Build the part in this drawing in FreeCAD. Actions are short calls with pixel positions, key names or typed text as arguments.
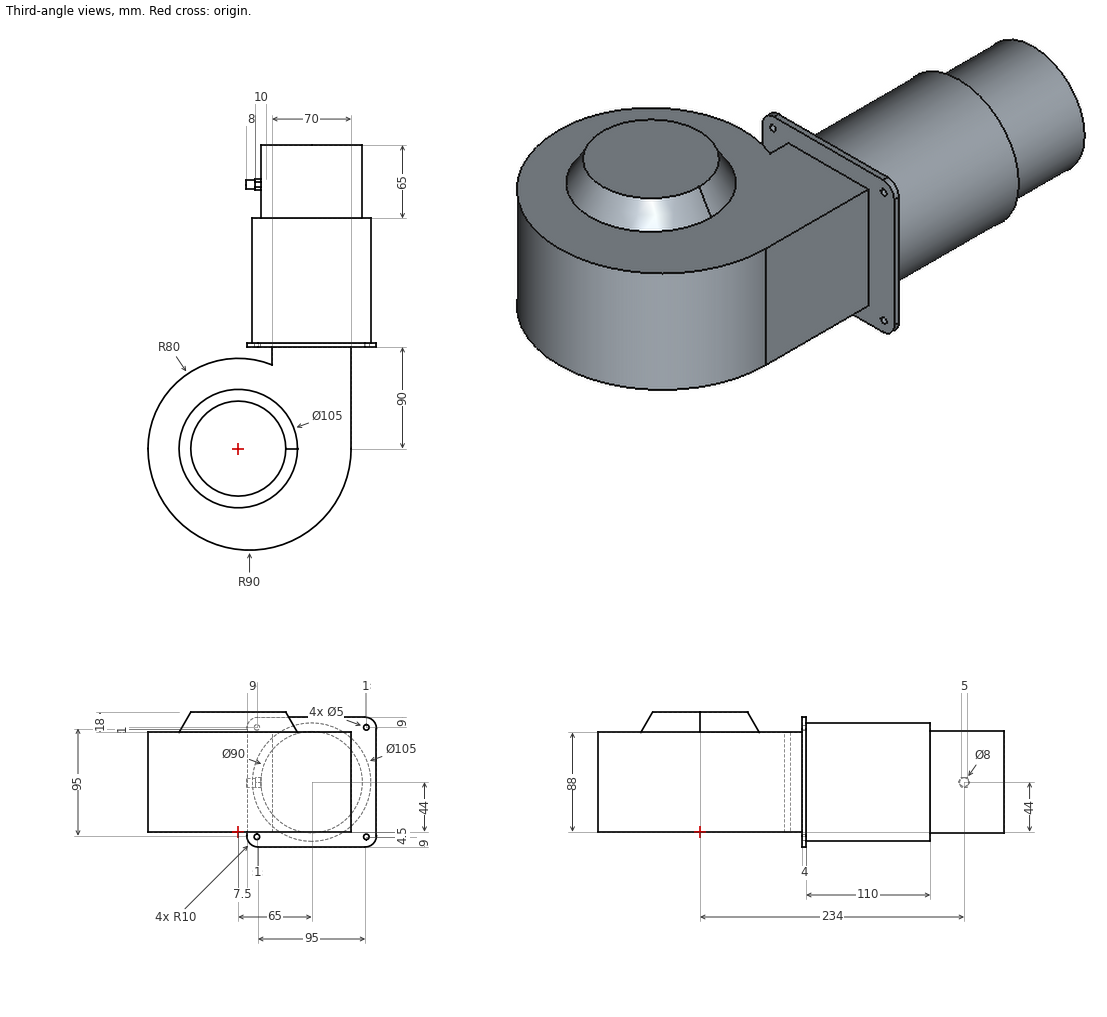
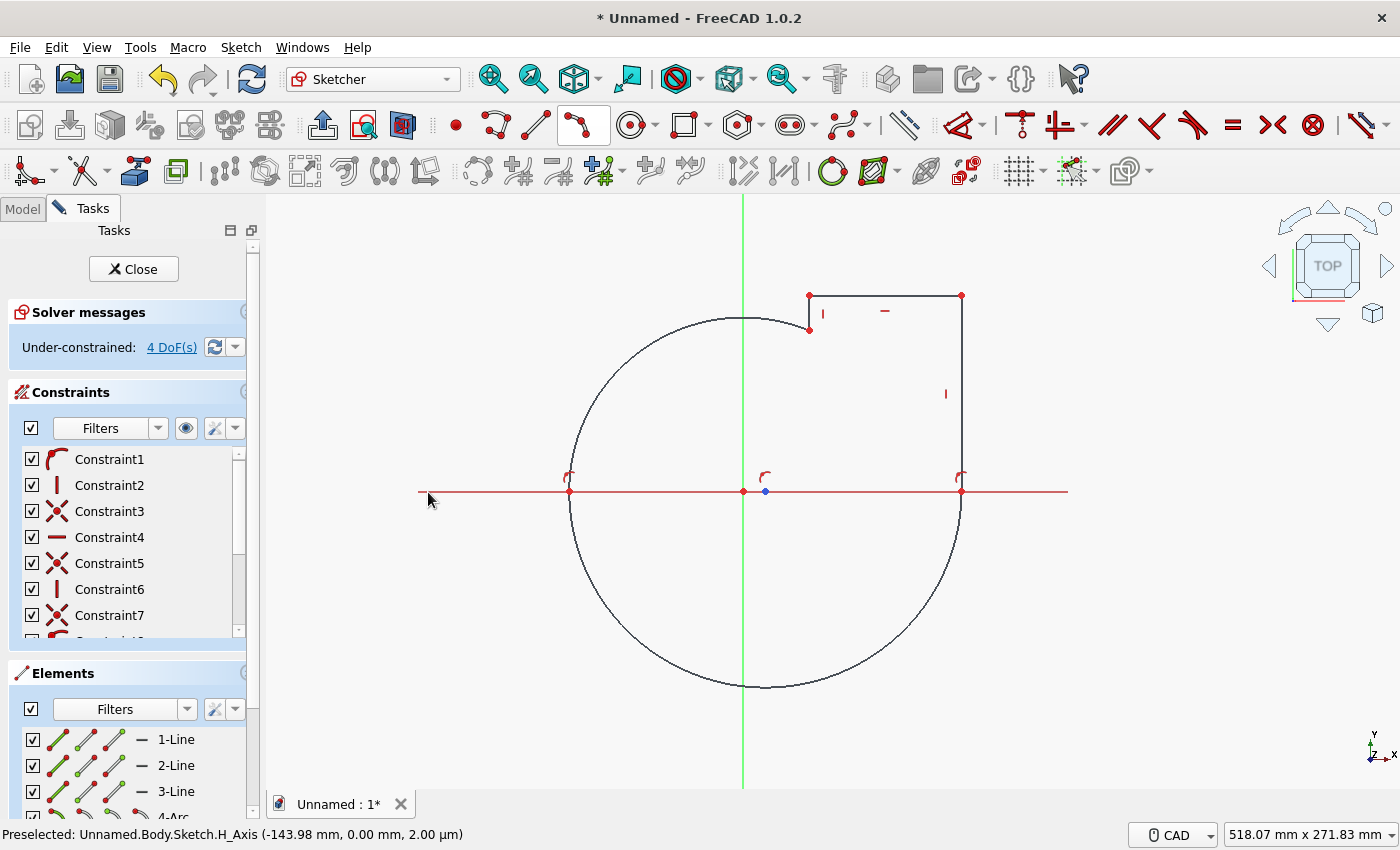
click(958, 126)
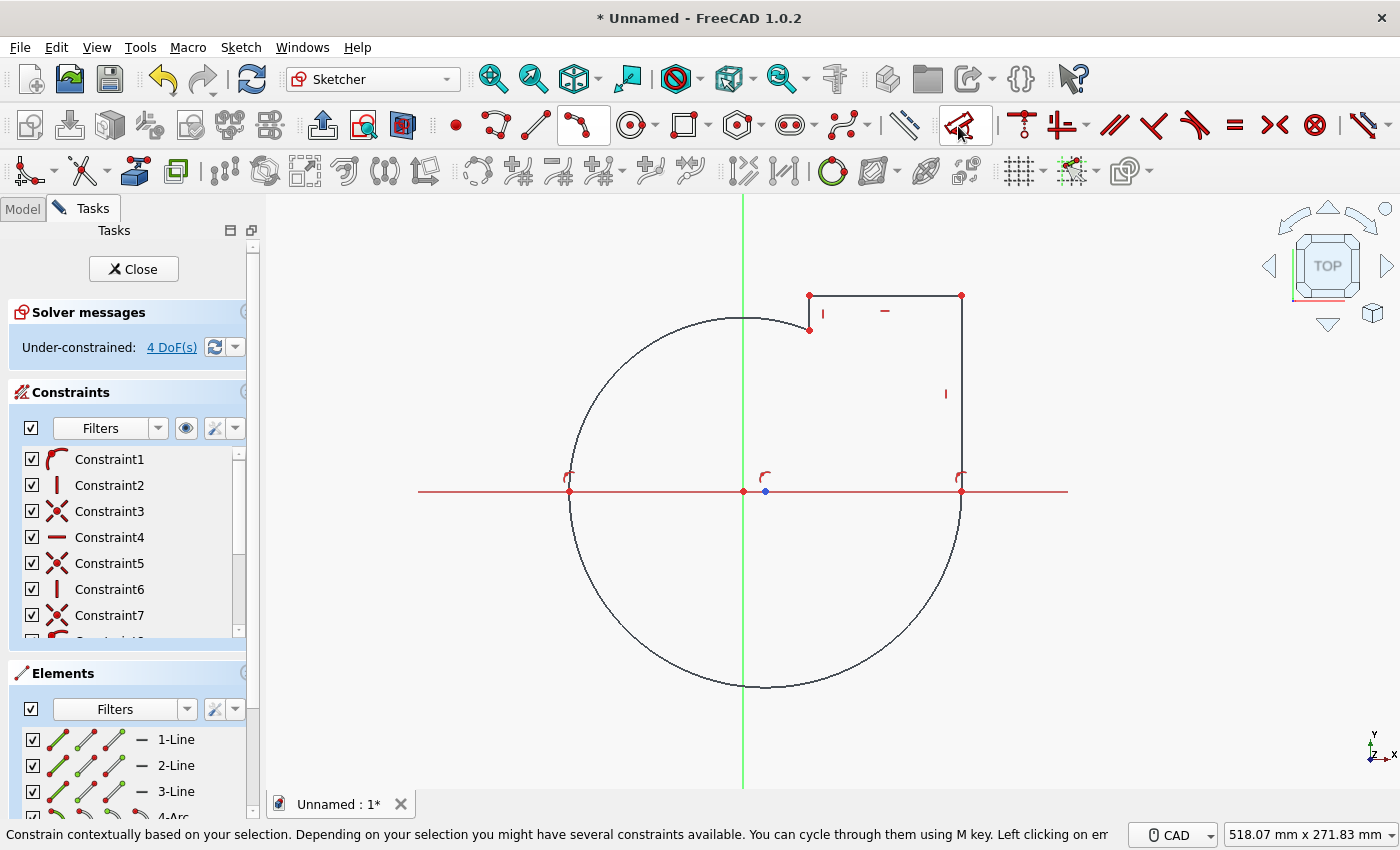
click(709, 321)
click(703, 290)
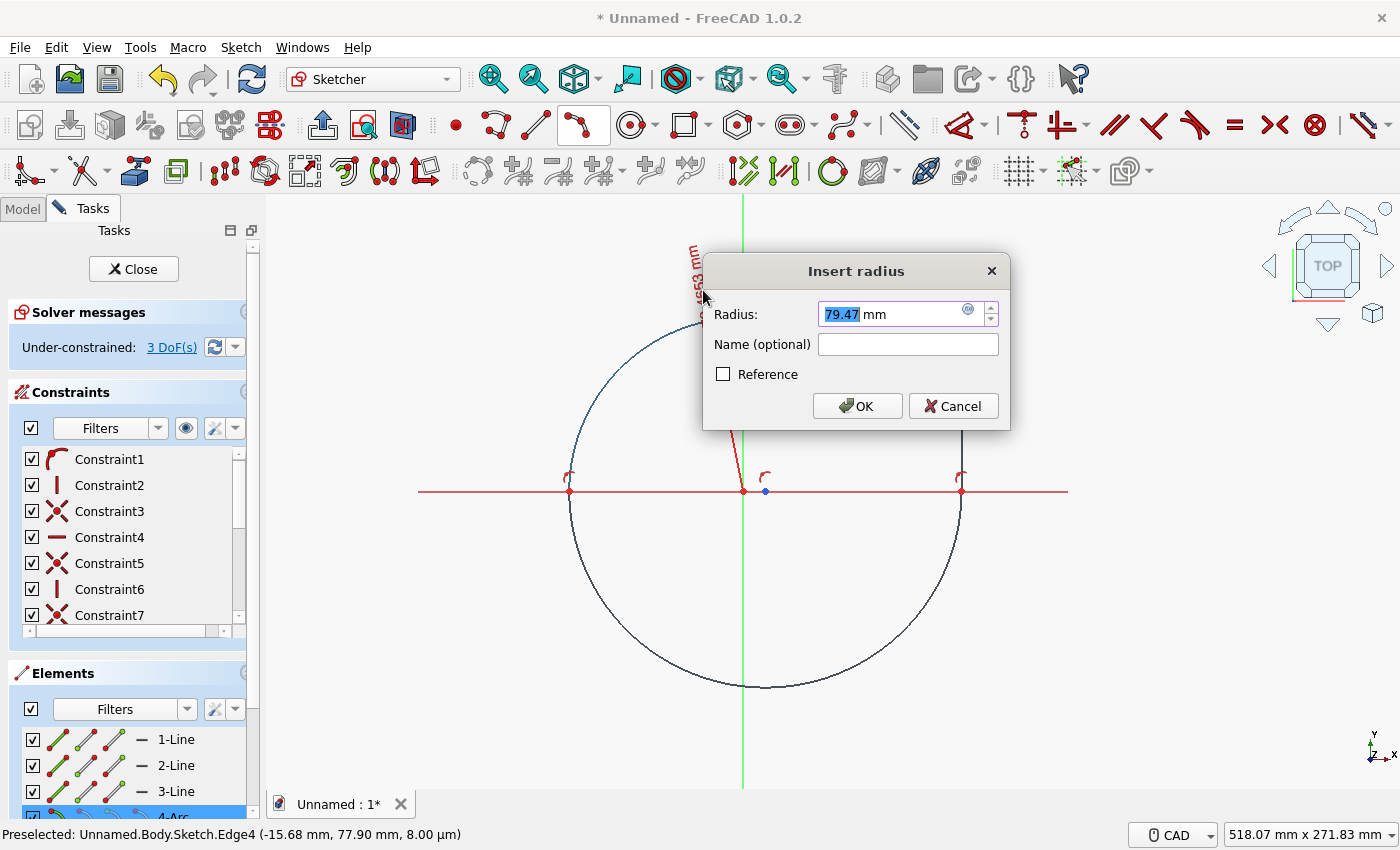
text(80)
key(Return)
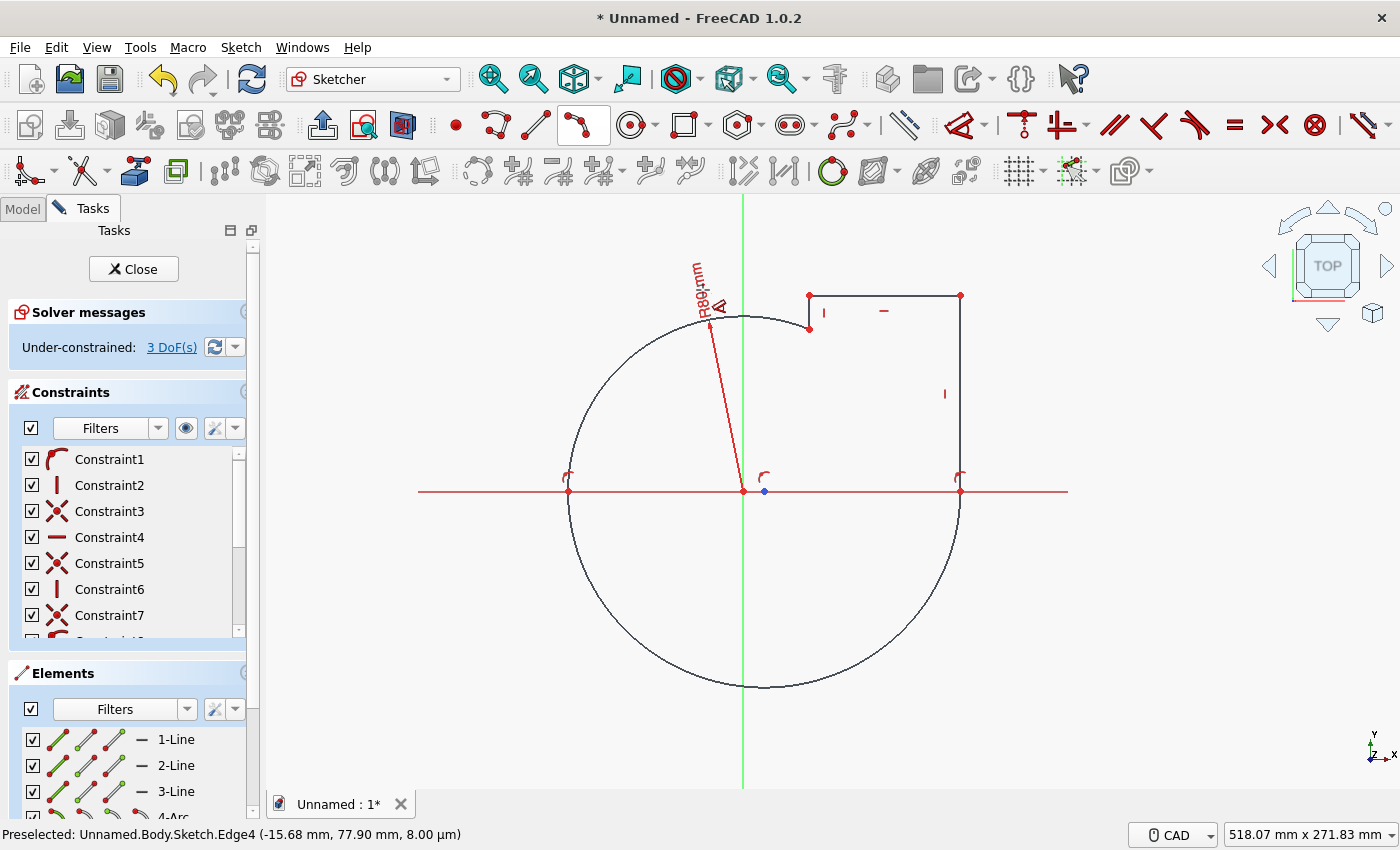
click(649, 650)
click(630, 676)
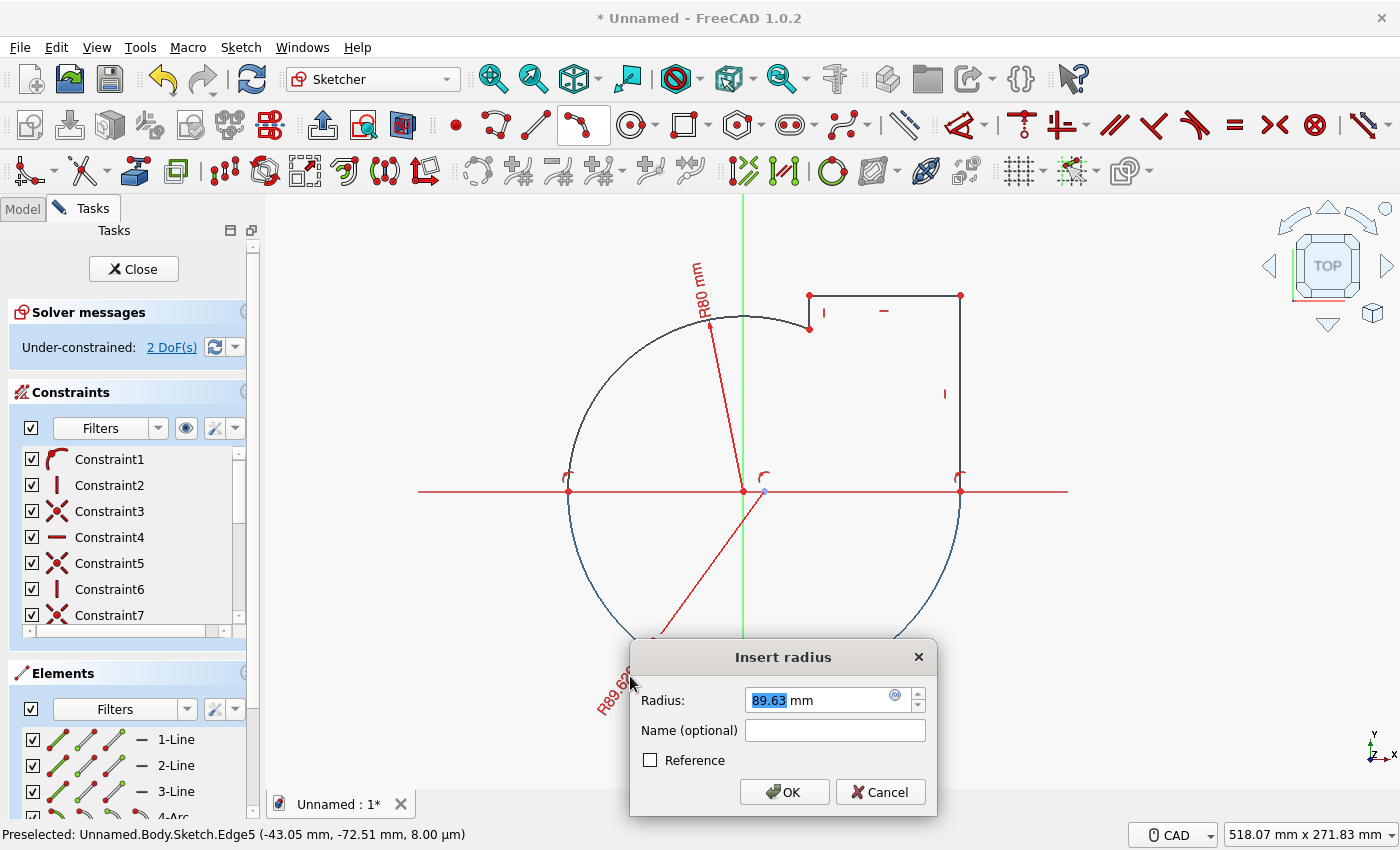
text(90)
key(Return)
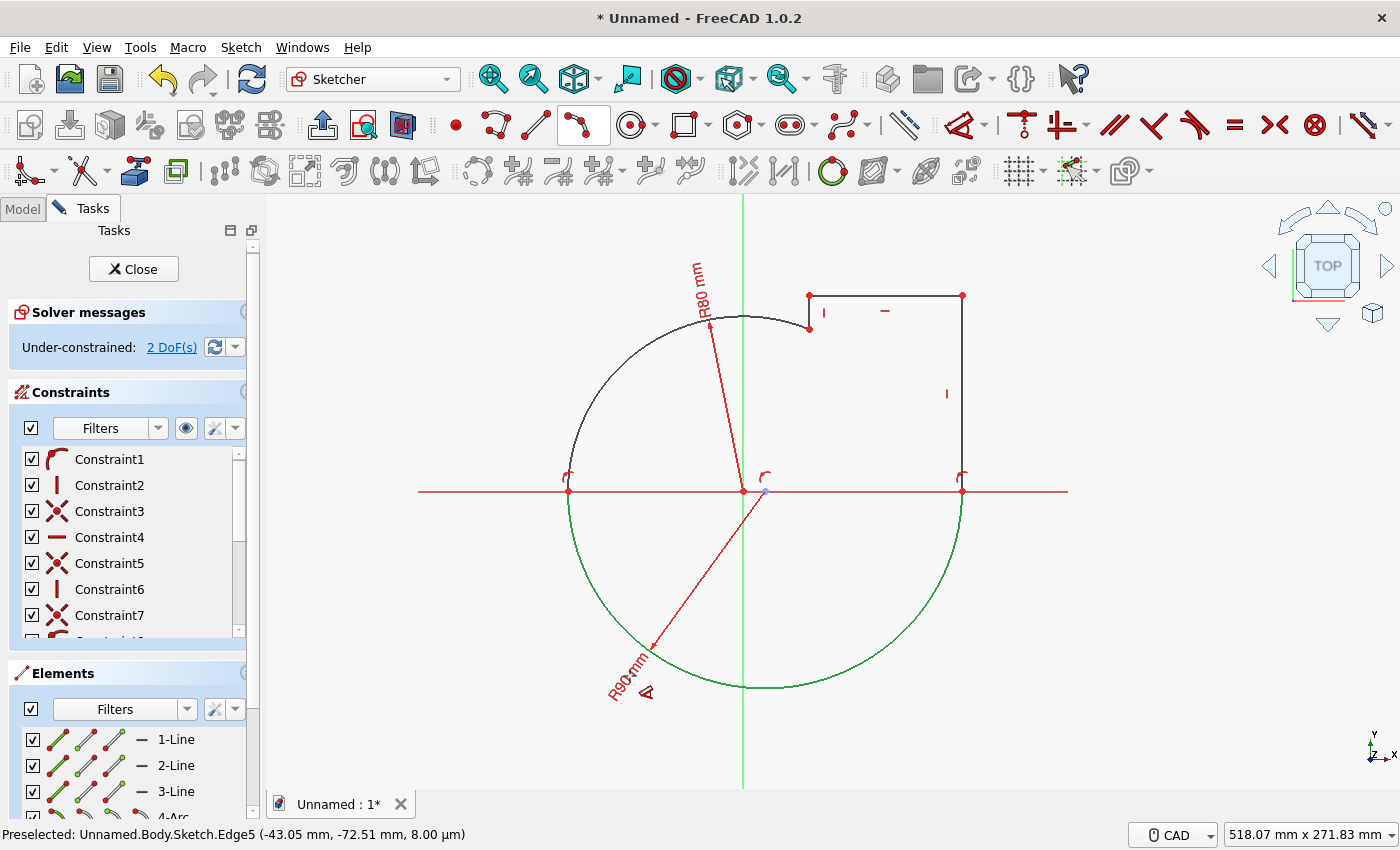
click(962, 433)
click(996, 394)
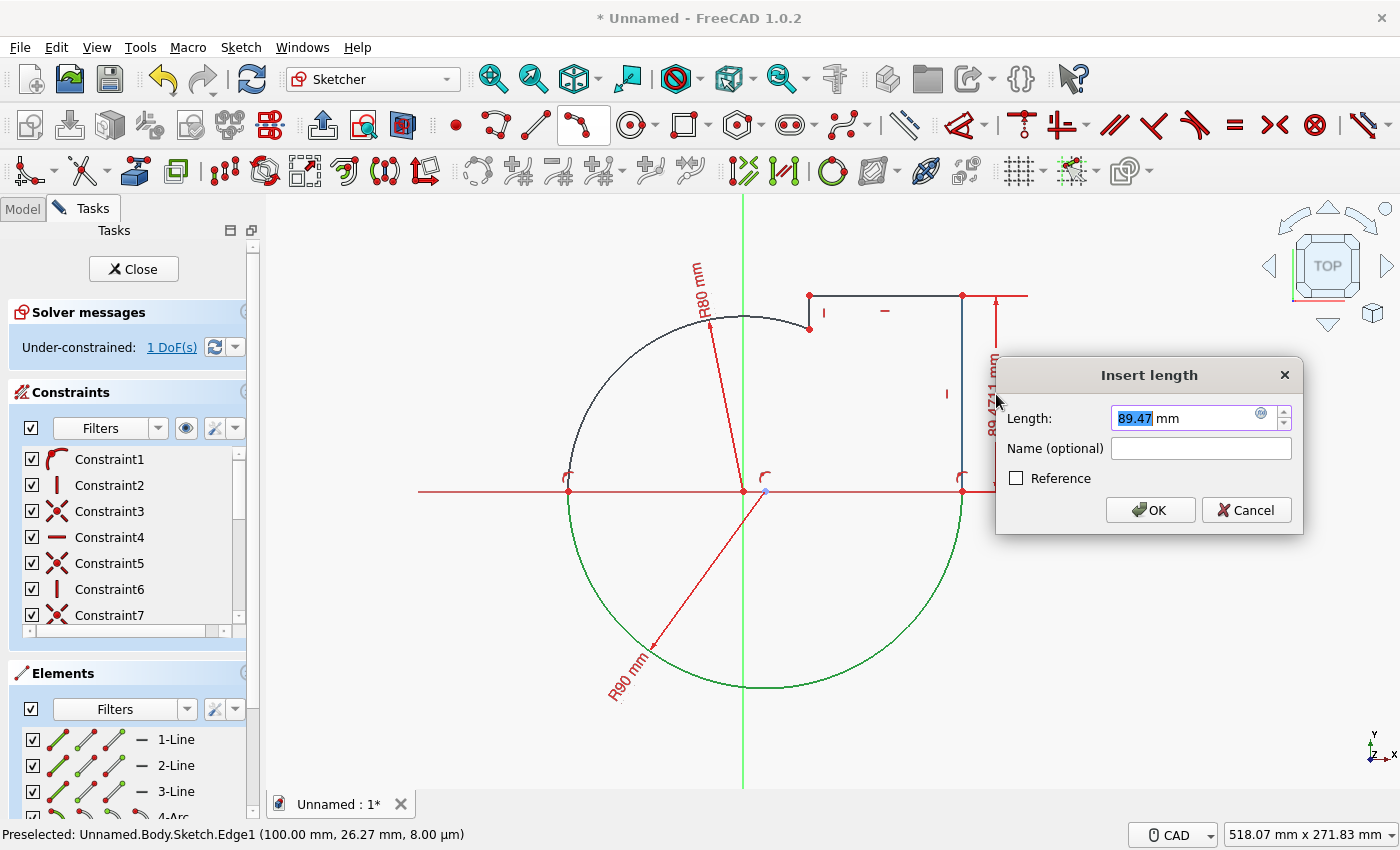
text(90)
key(Return)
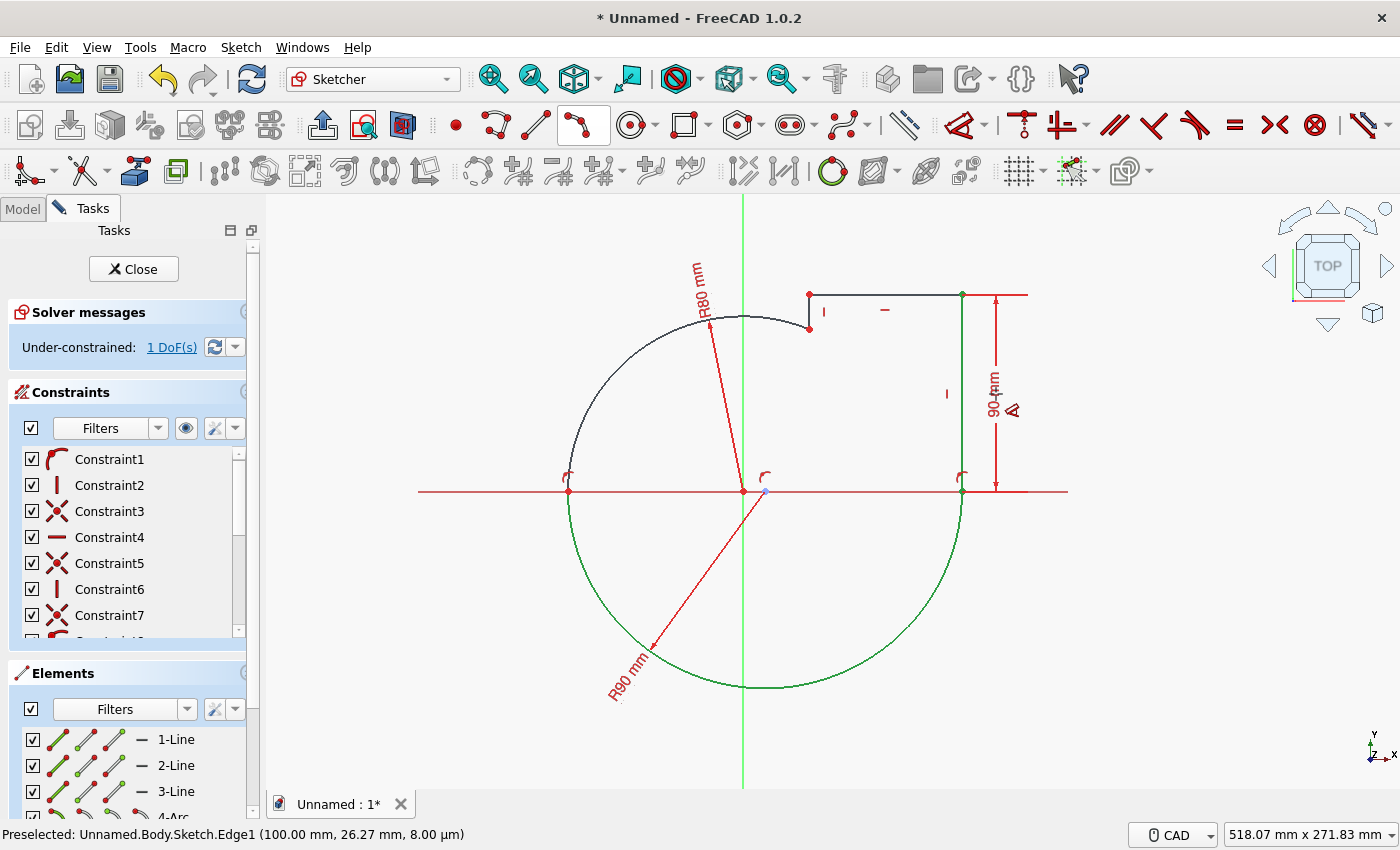
click(916, 295)
click(886, 261)